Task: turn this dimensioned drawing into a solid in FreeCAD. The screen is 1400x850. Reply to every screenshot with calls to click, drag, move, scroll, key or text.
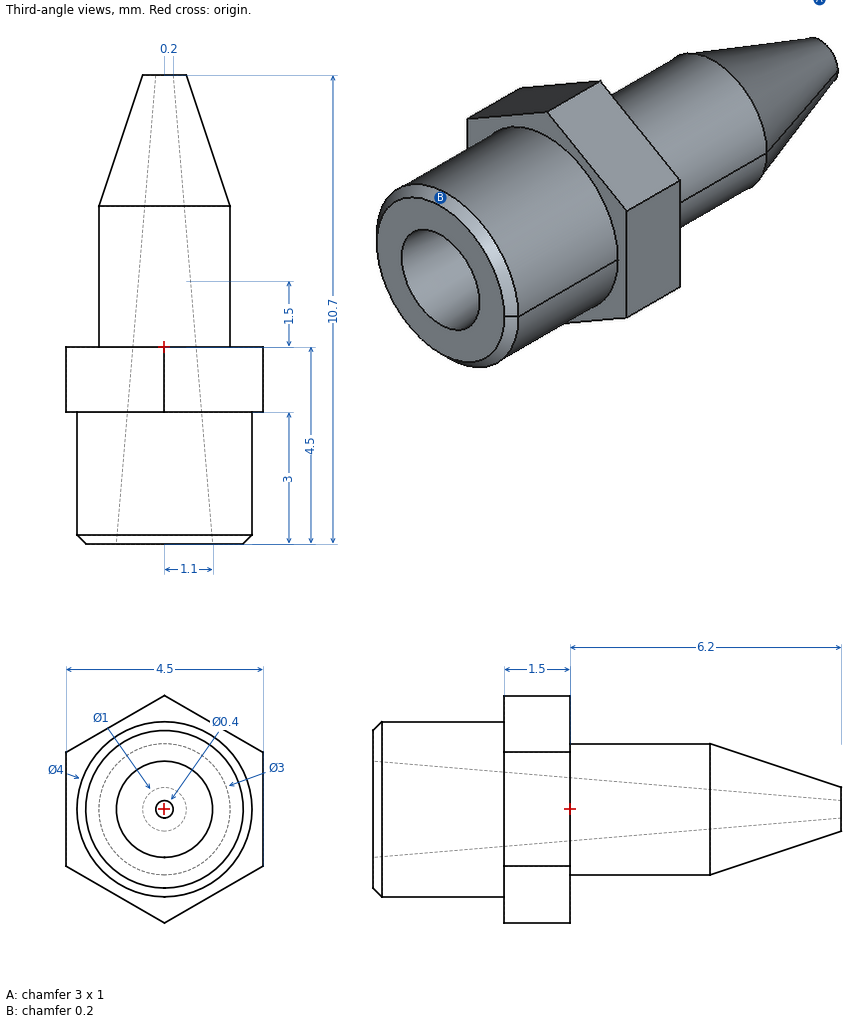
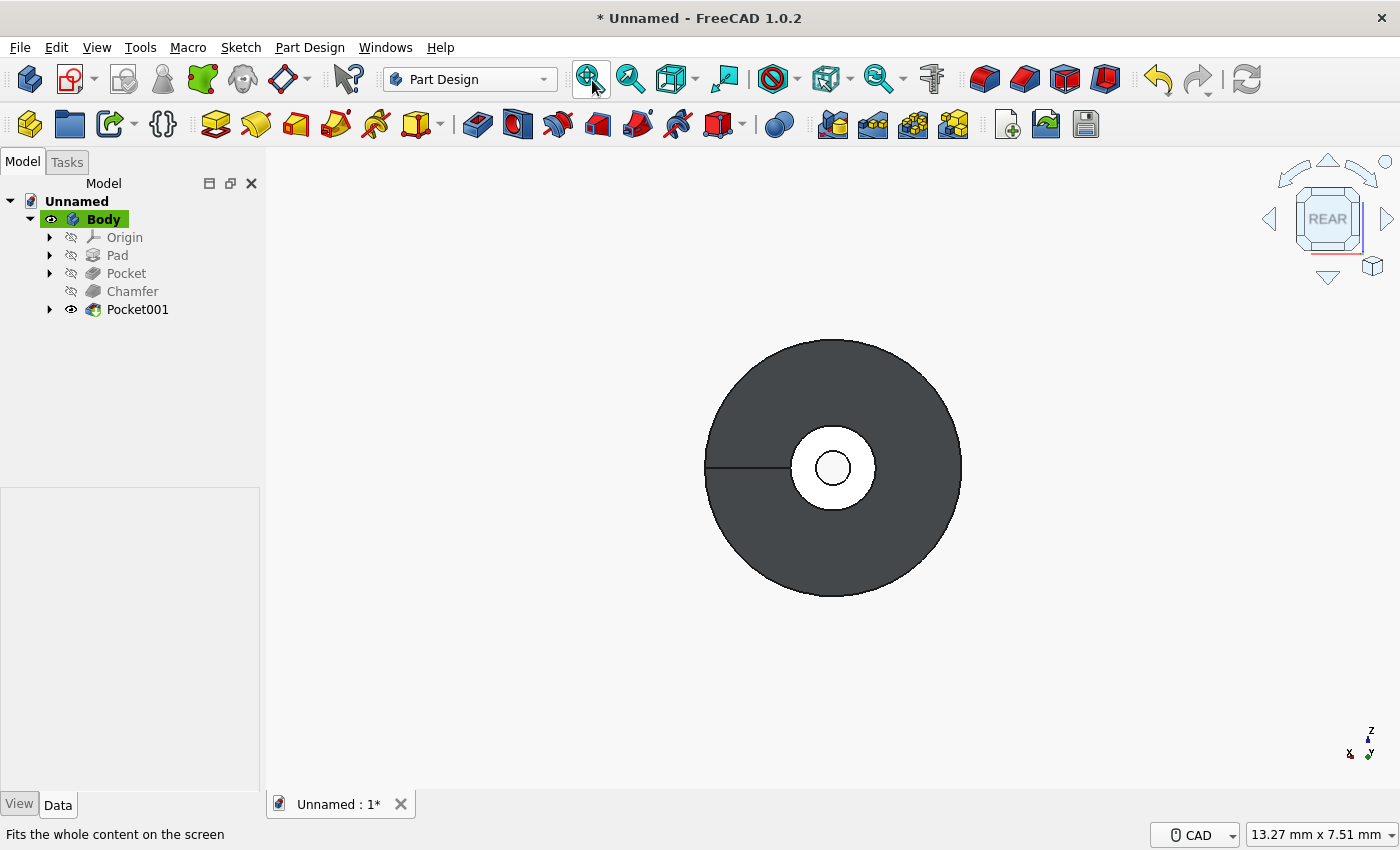
click(50, 237)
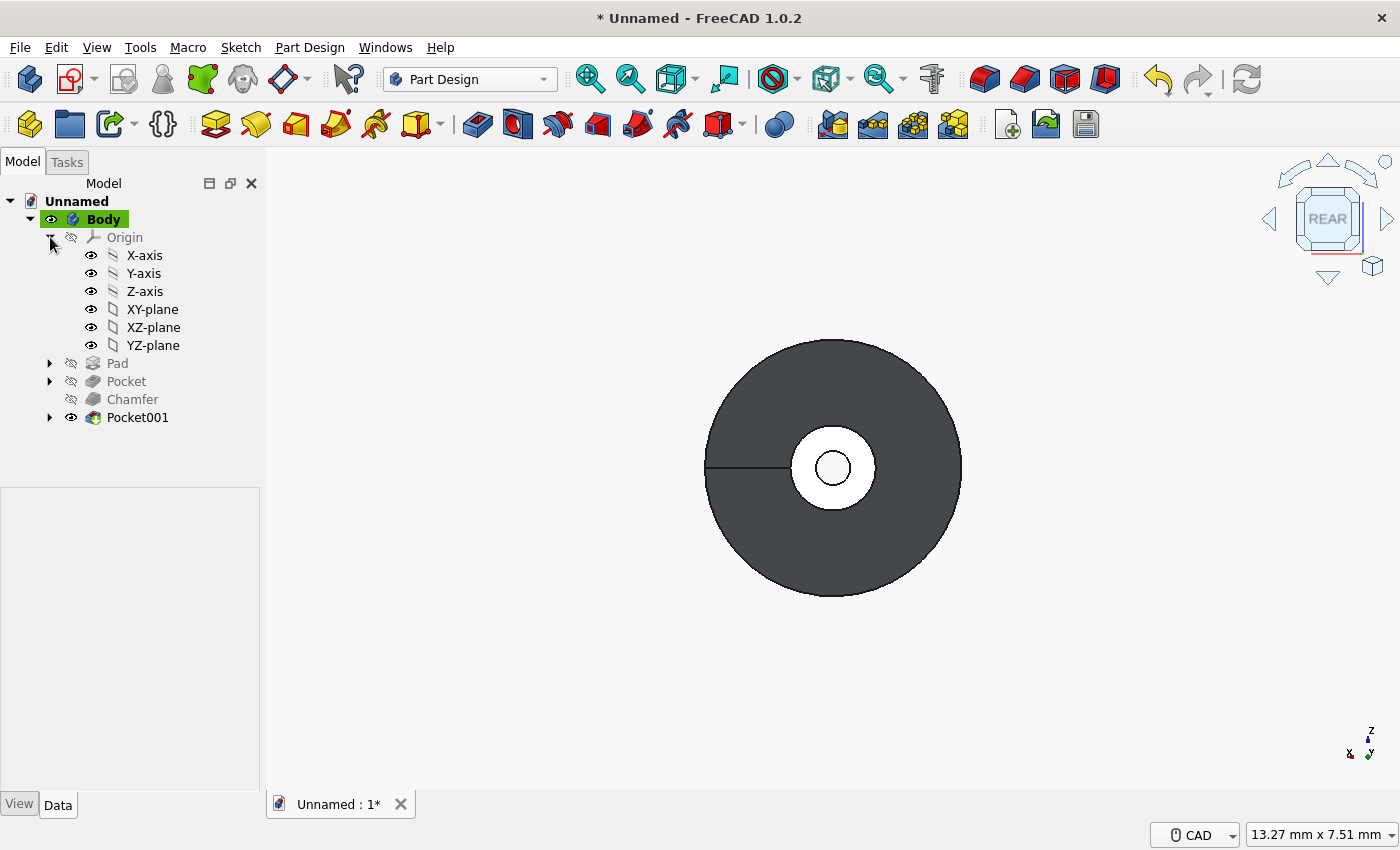
click(136, 327)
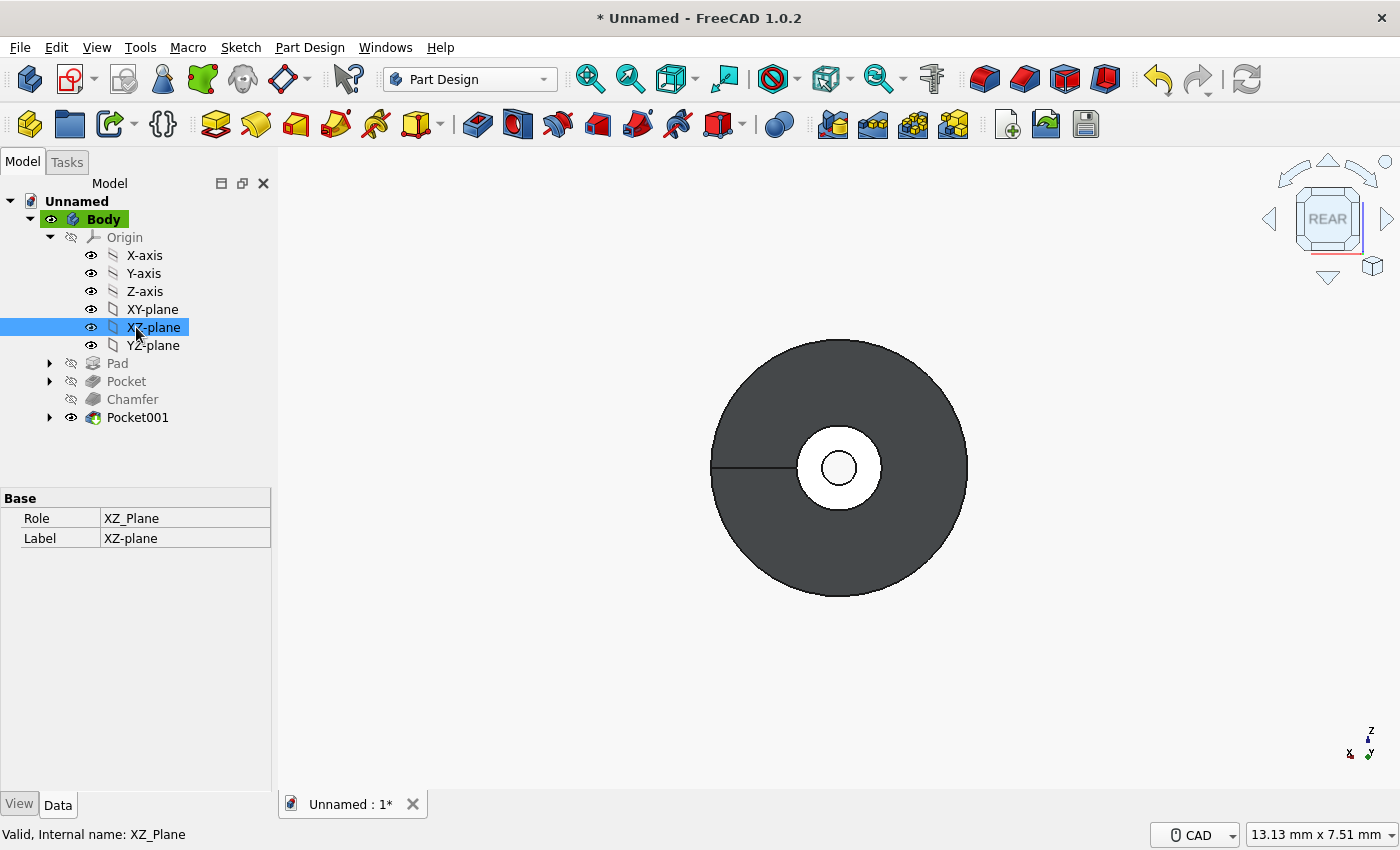
click(284, 80)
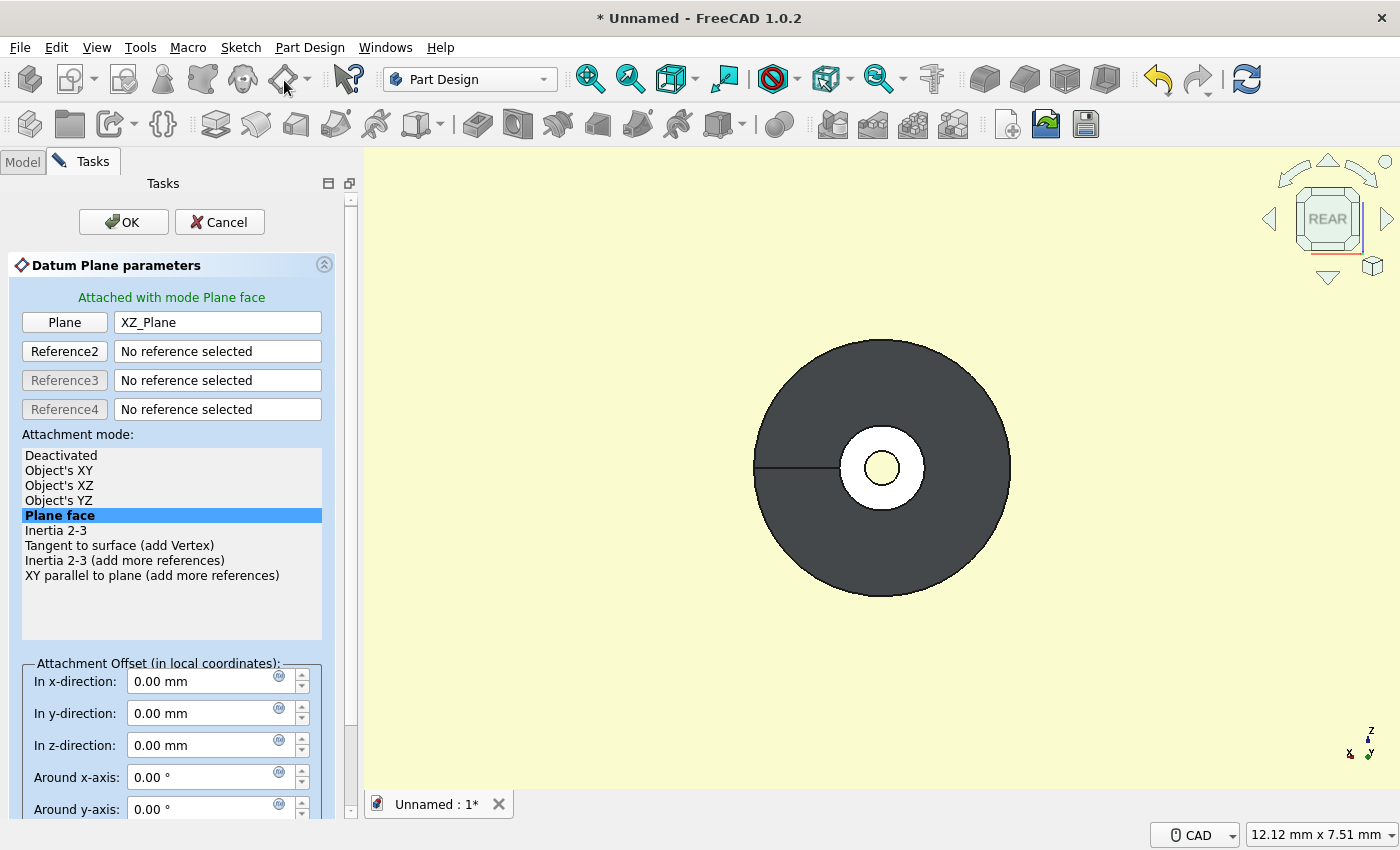
triple_click(210, 745)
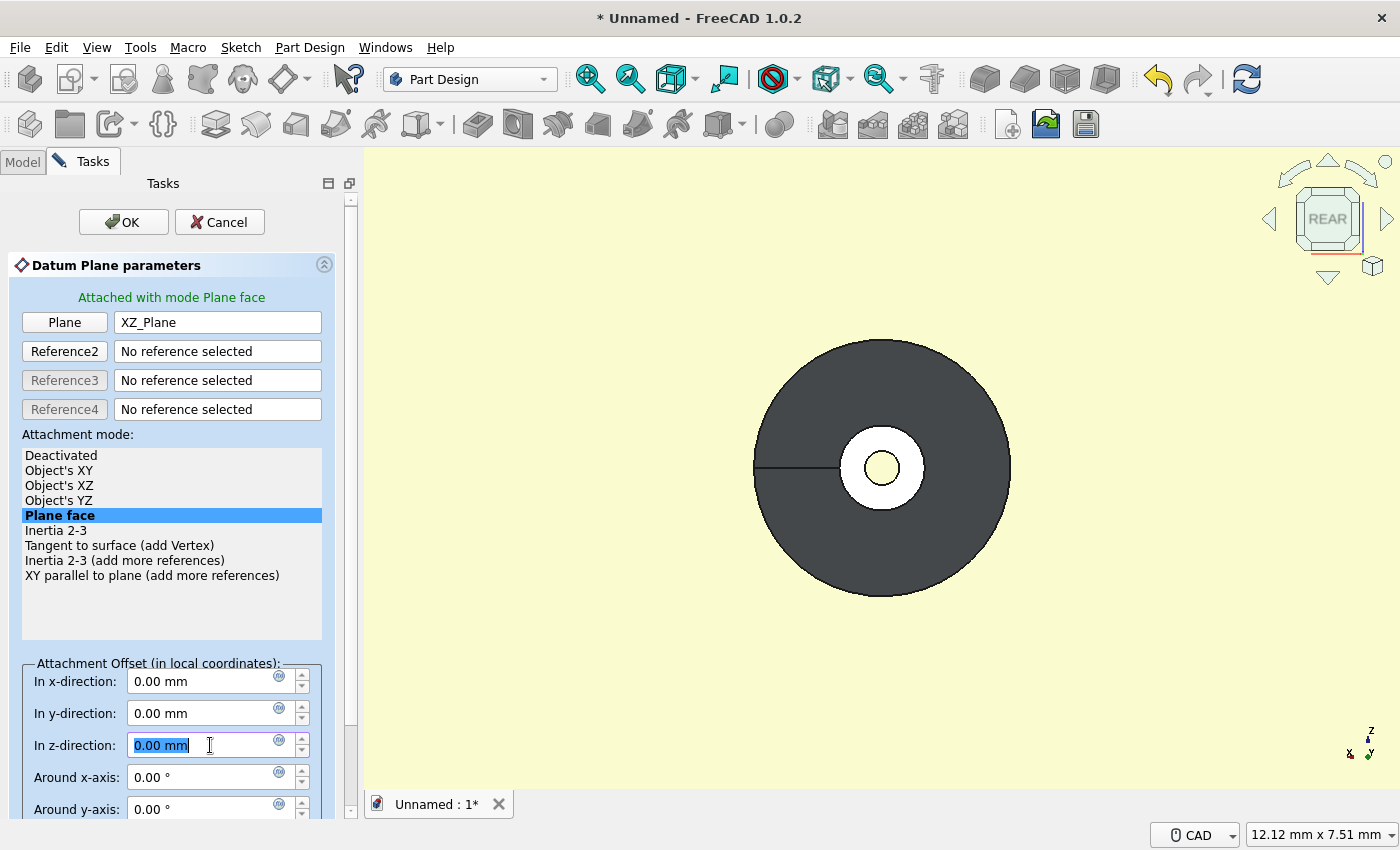
text(1.5)
key(Tab)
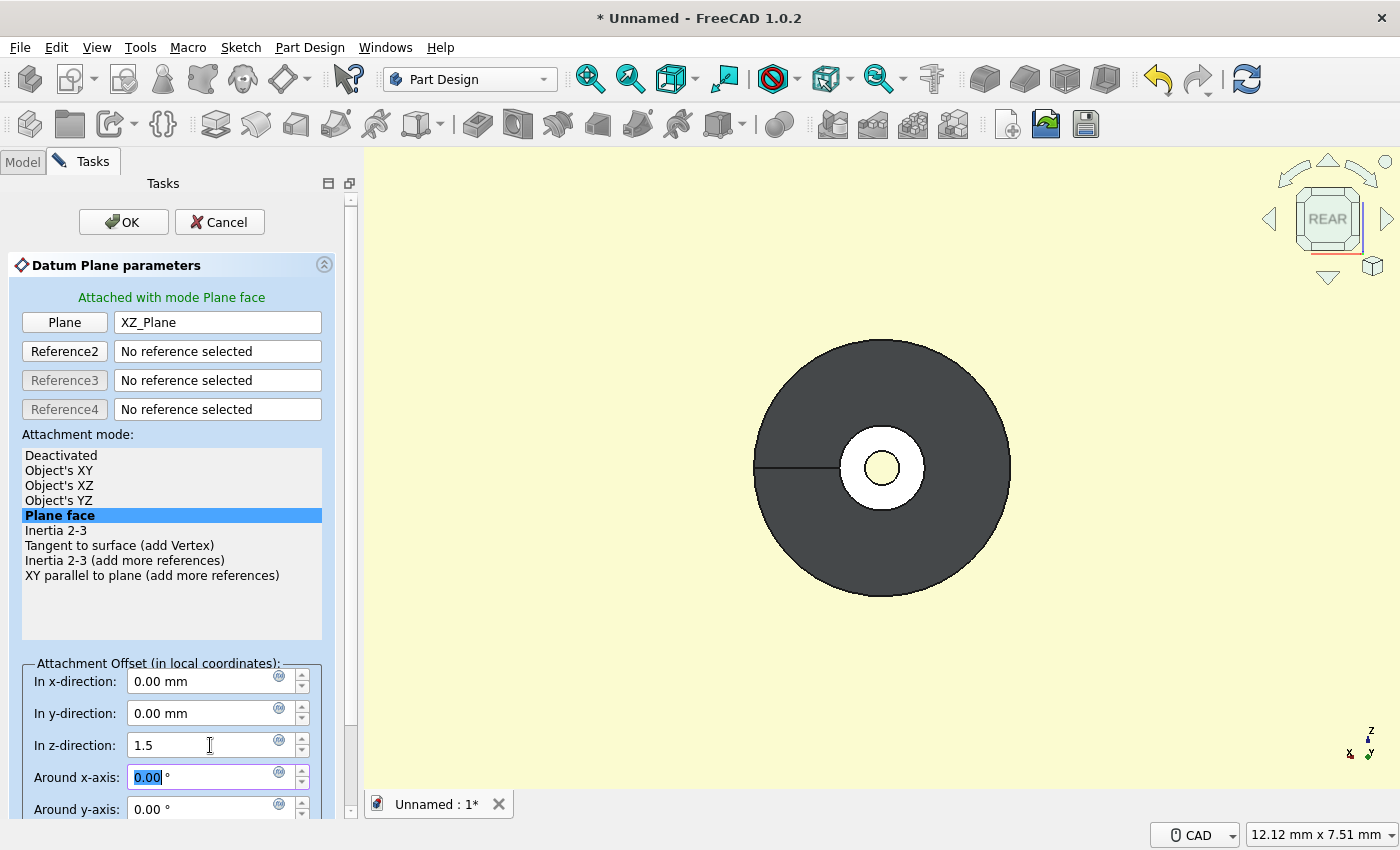
click(124, 222)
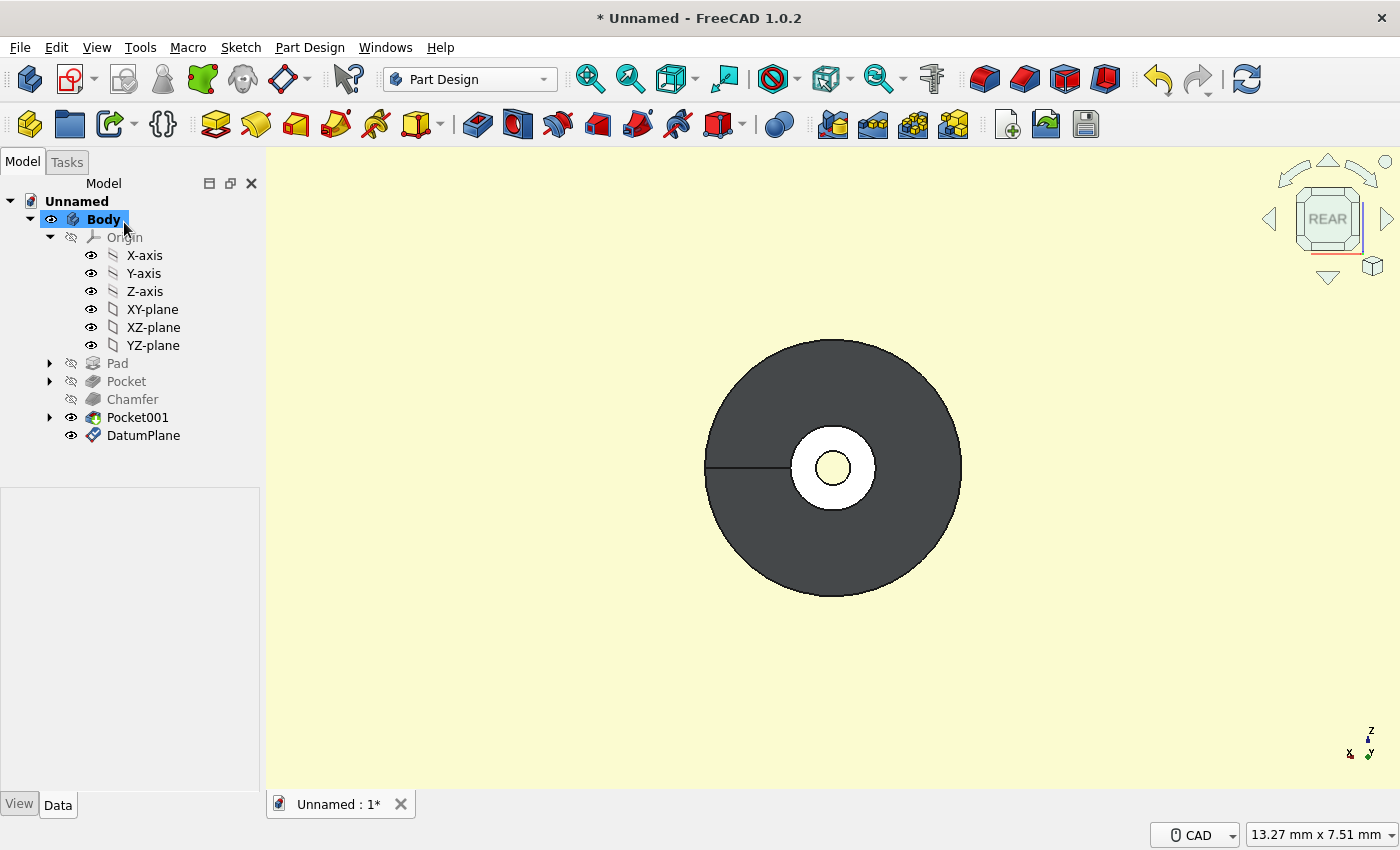
click(116, 435)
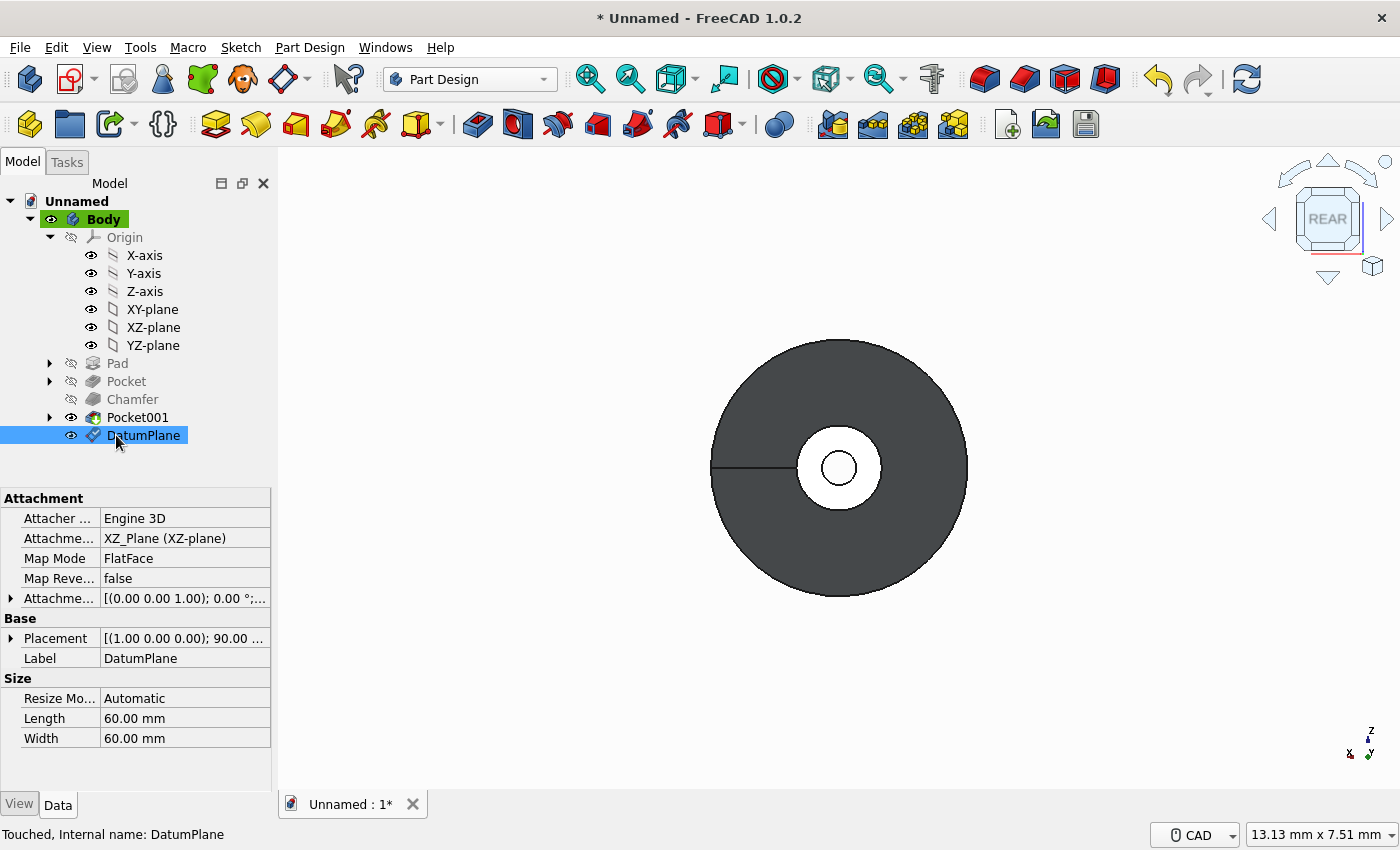
click(70, 80)